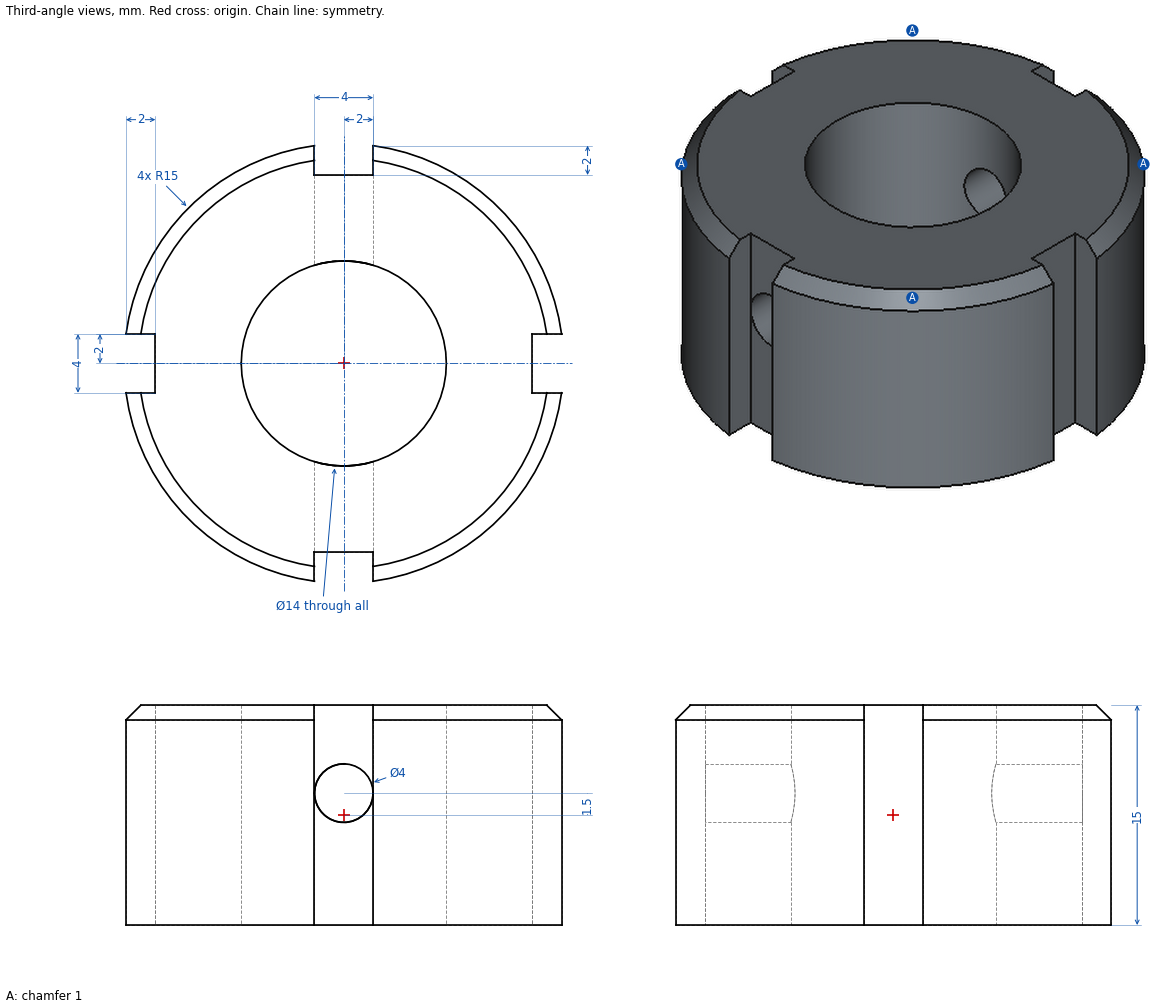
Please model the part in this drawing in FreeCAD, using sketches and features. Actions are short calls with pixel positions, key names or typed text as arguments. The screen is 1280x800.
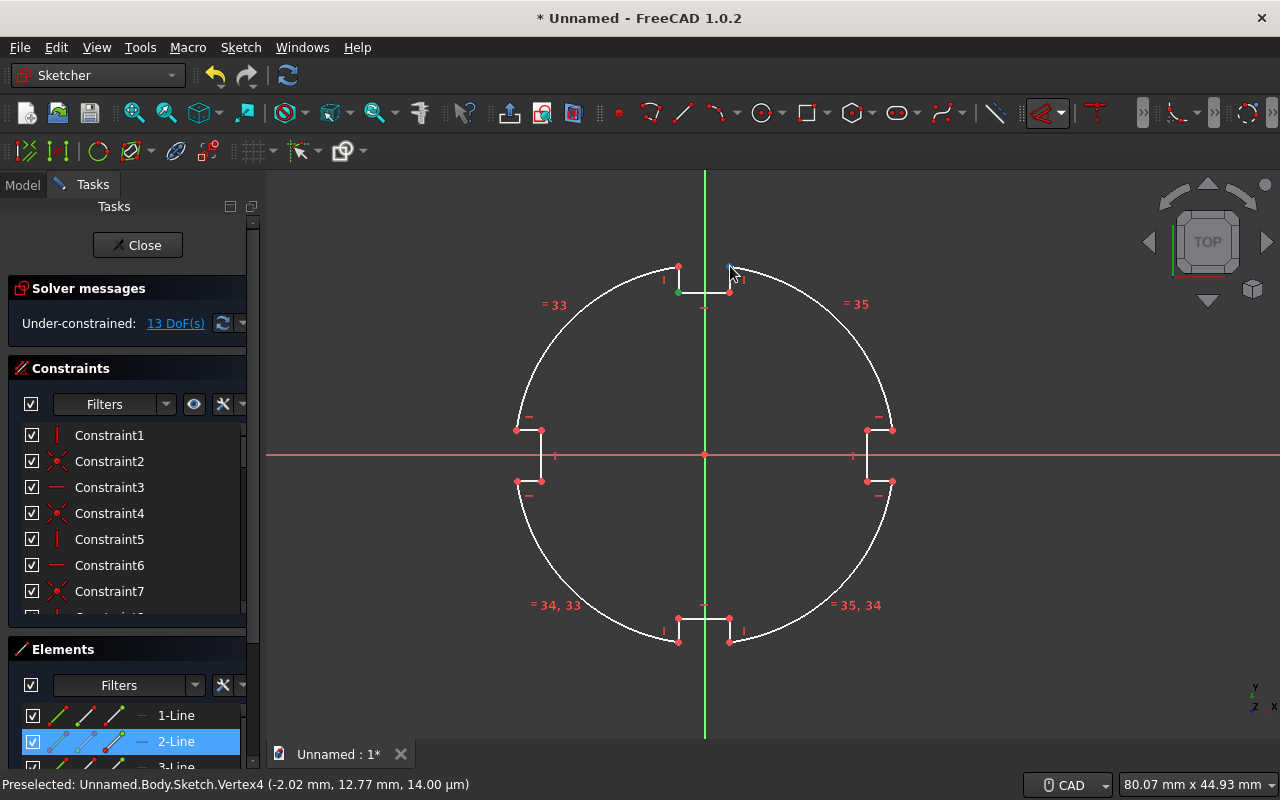
click(679, 619)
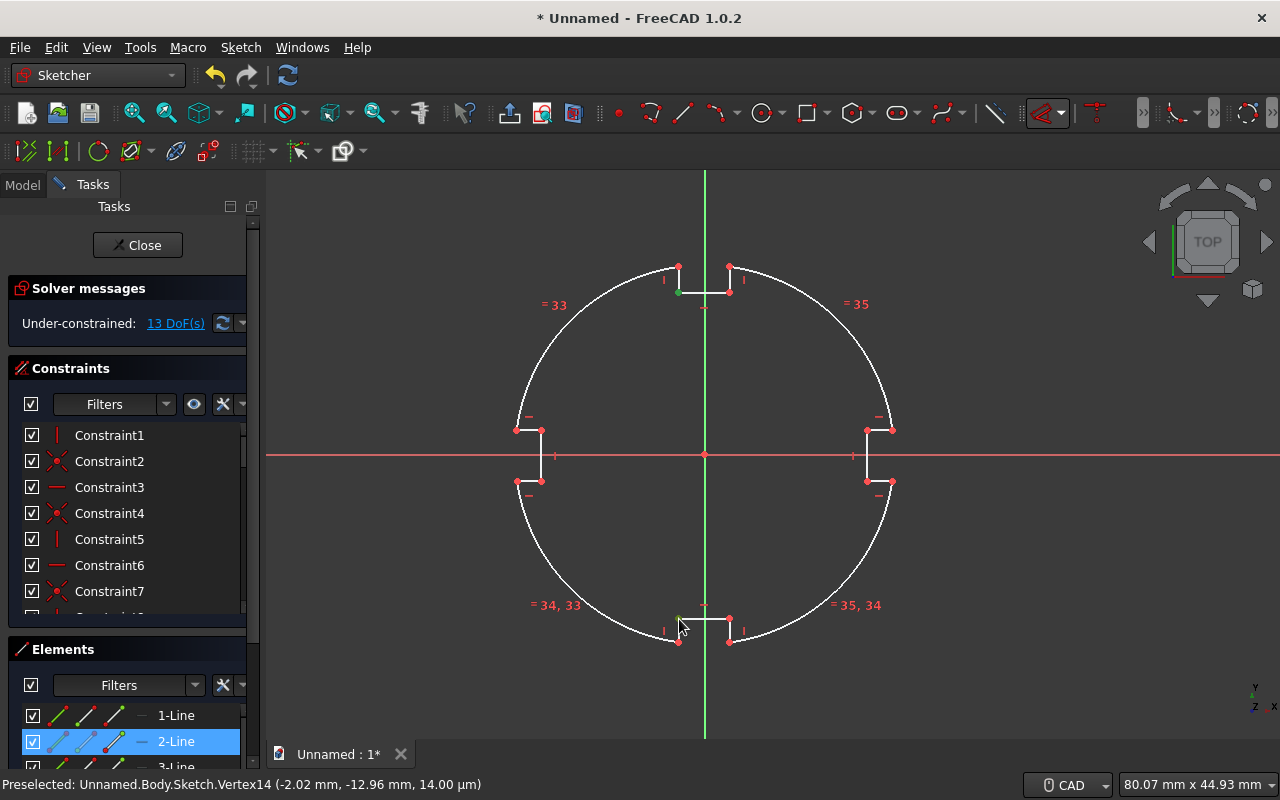
click(353, 455)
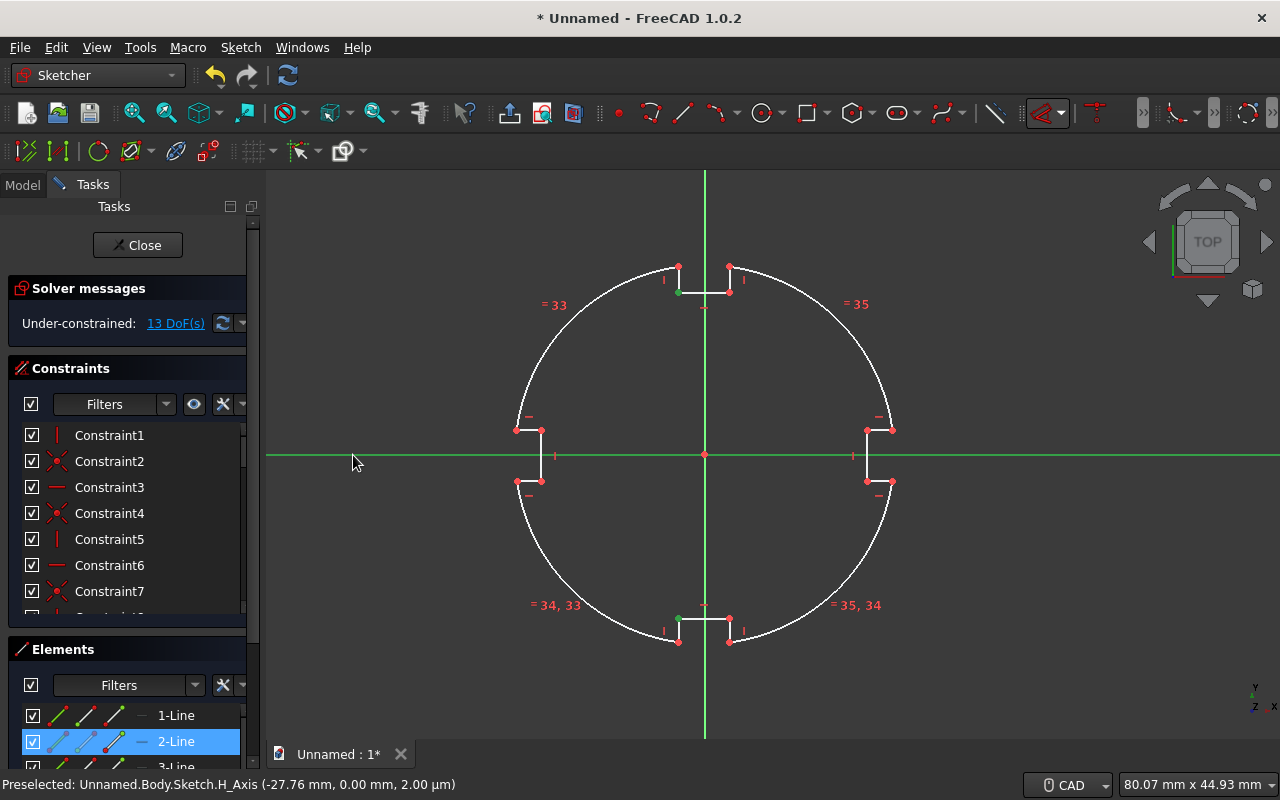
key(s)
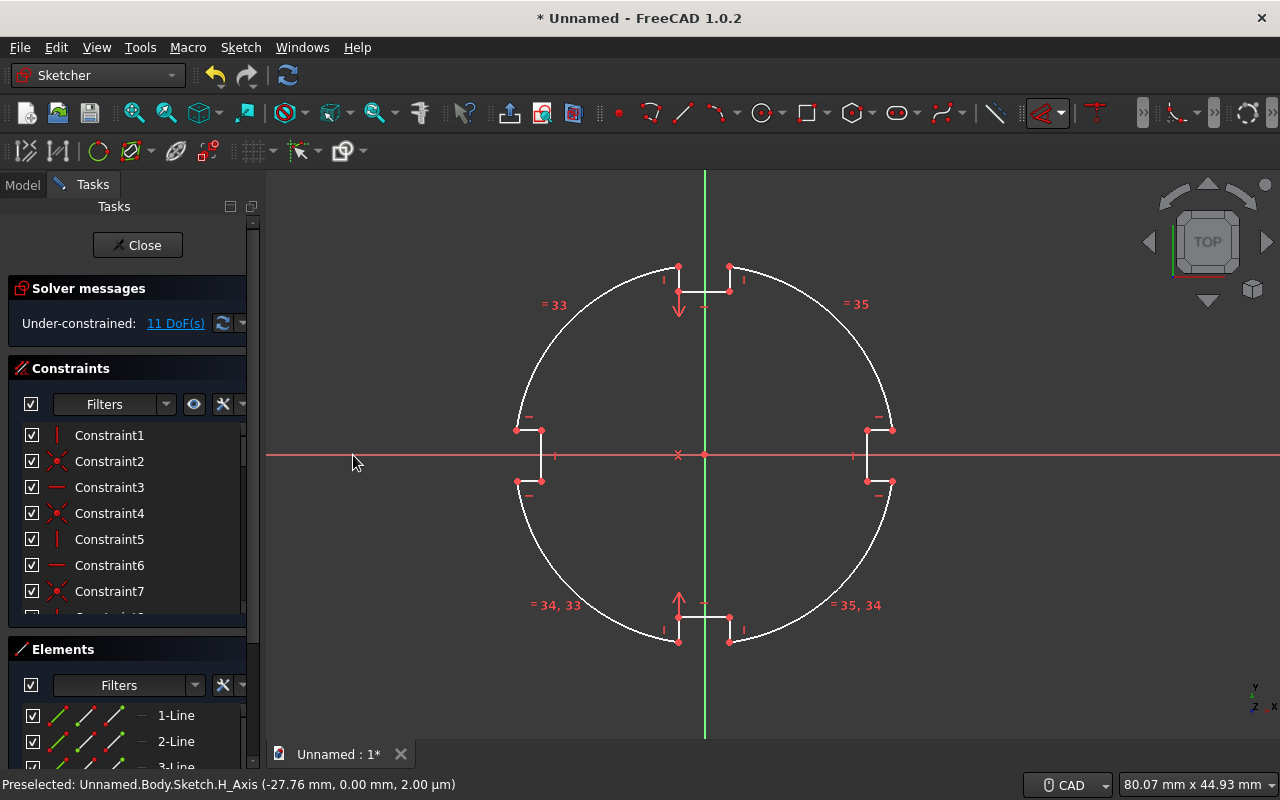
click(541, 481)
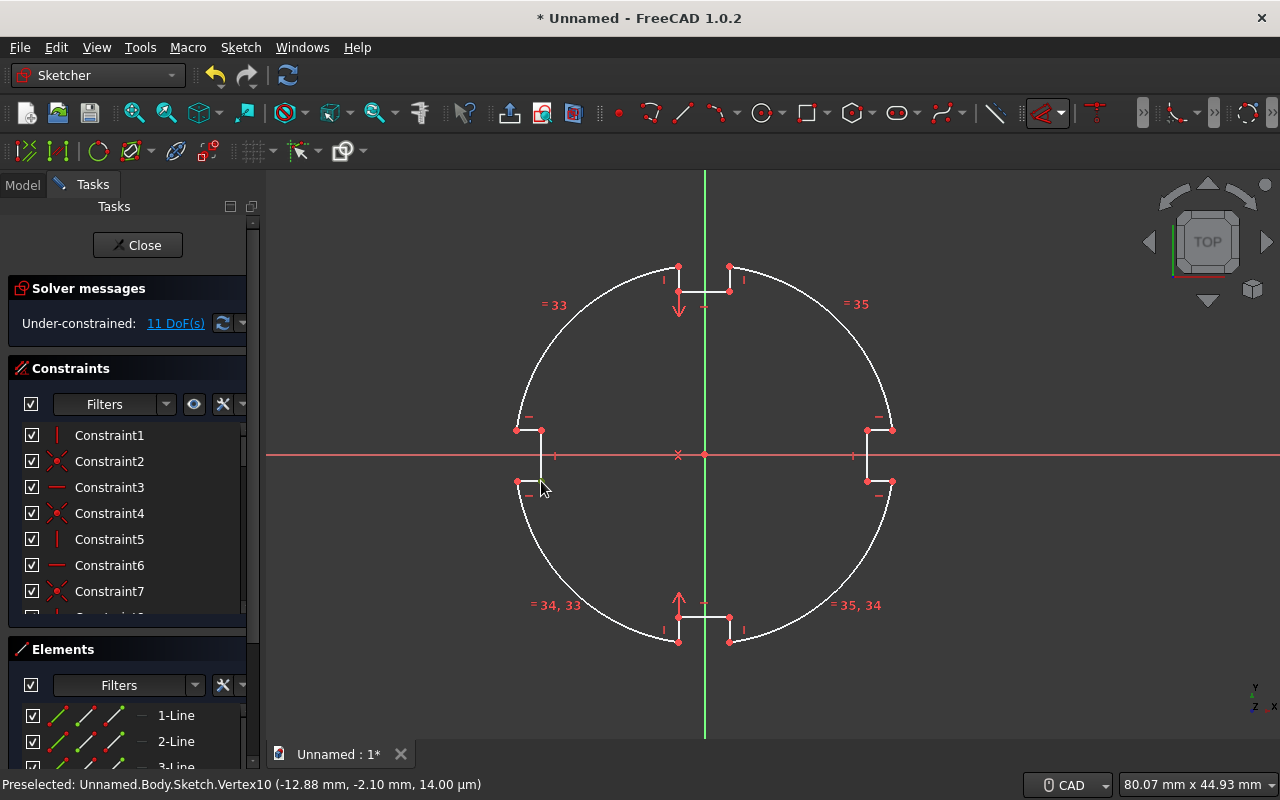
click(867, 481)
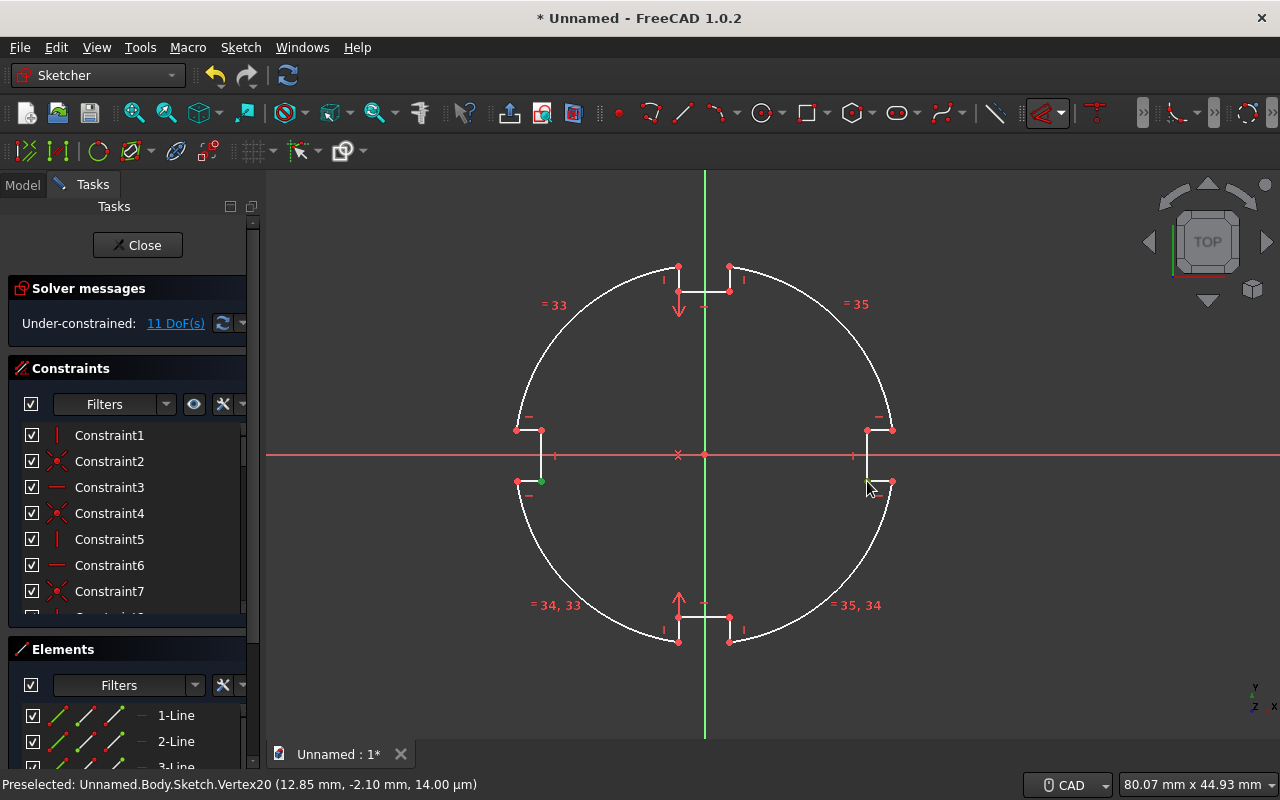
click(705, 674)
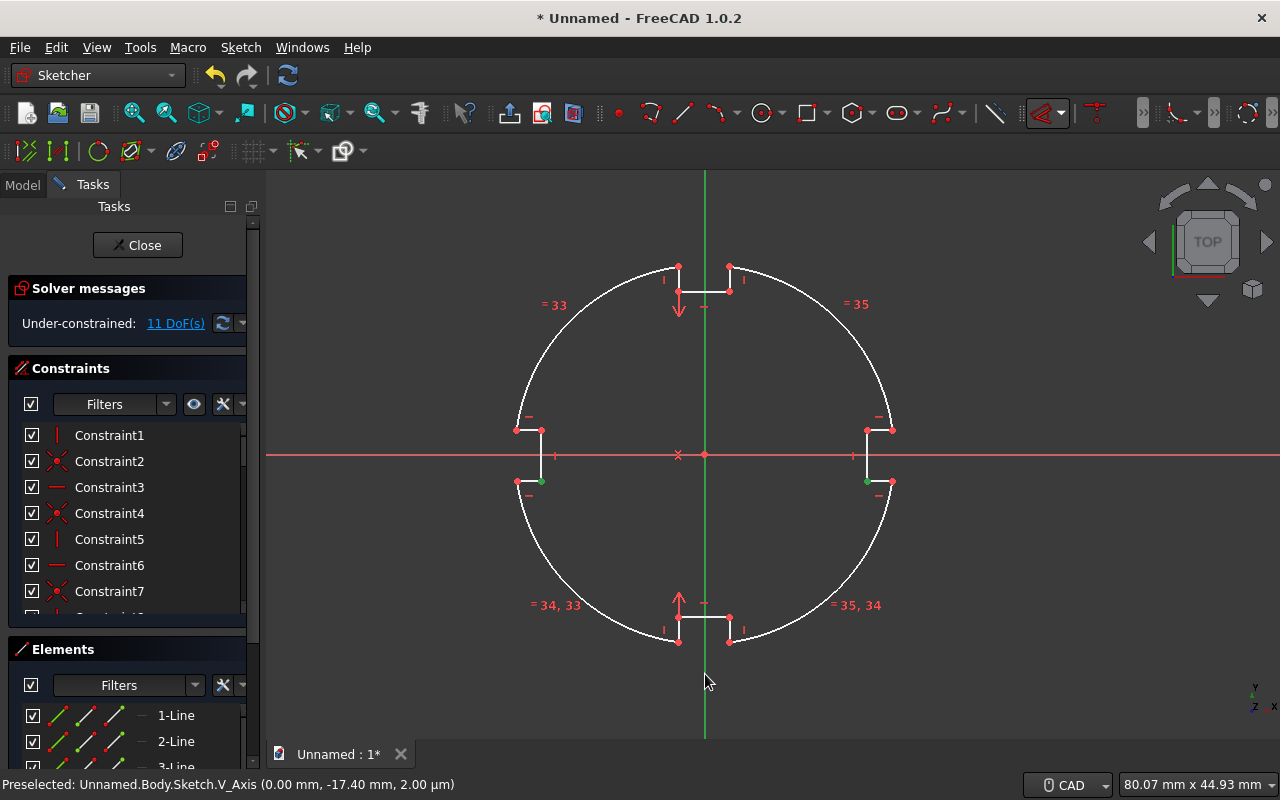
key(s)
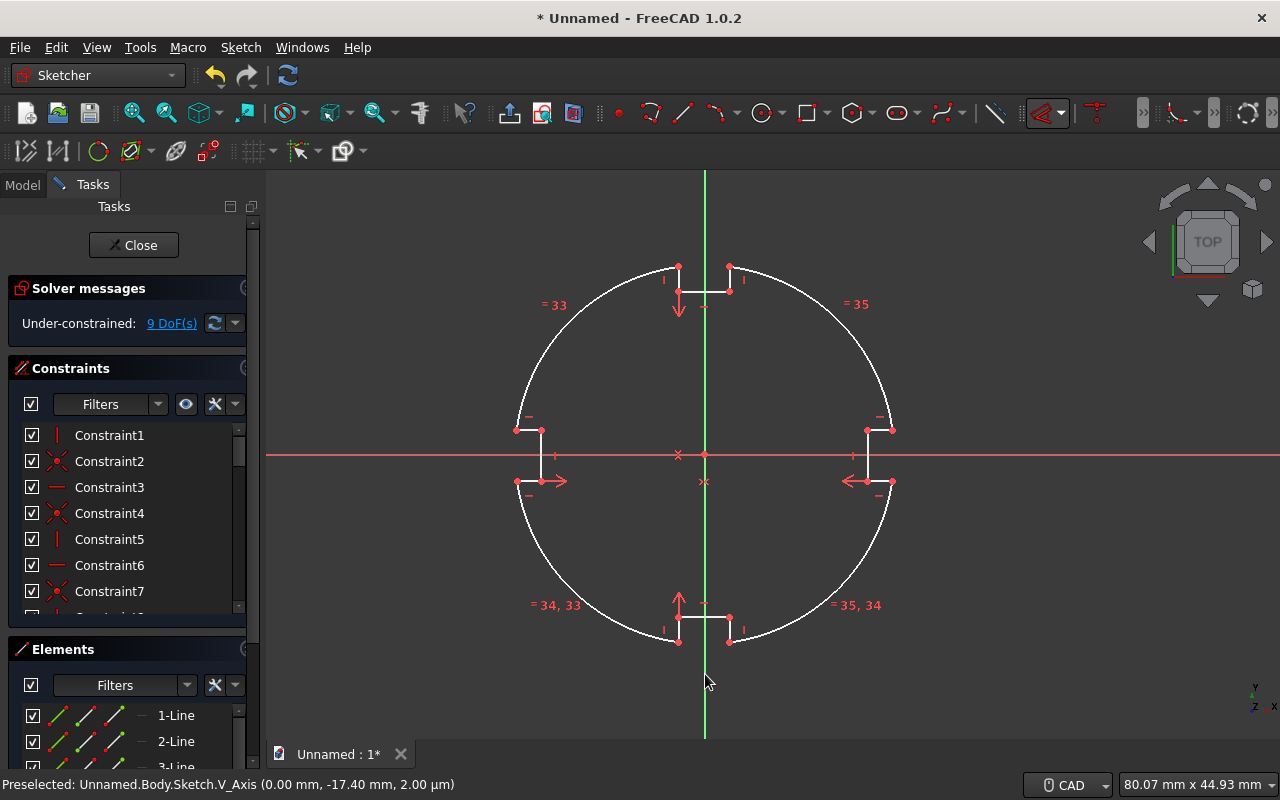
click(609, 291)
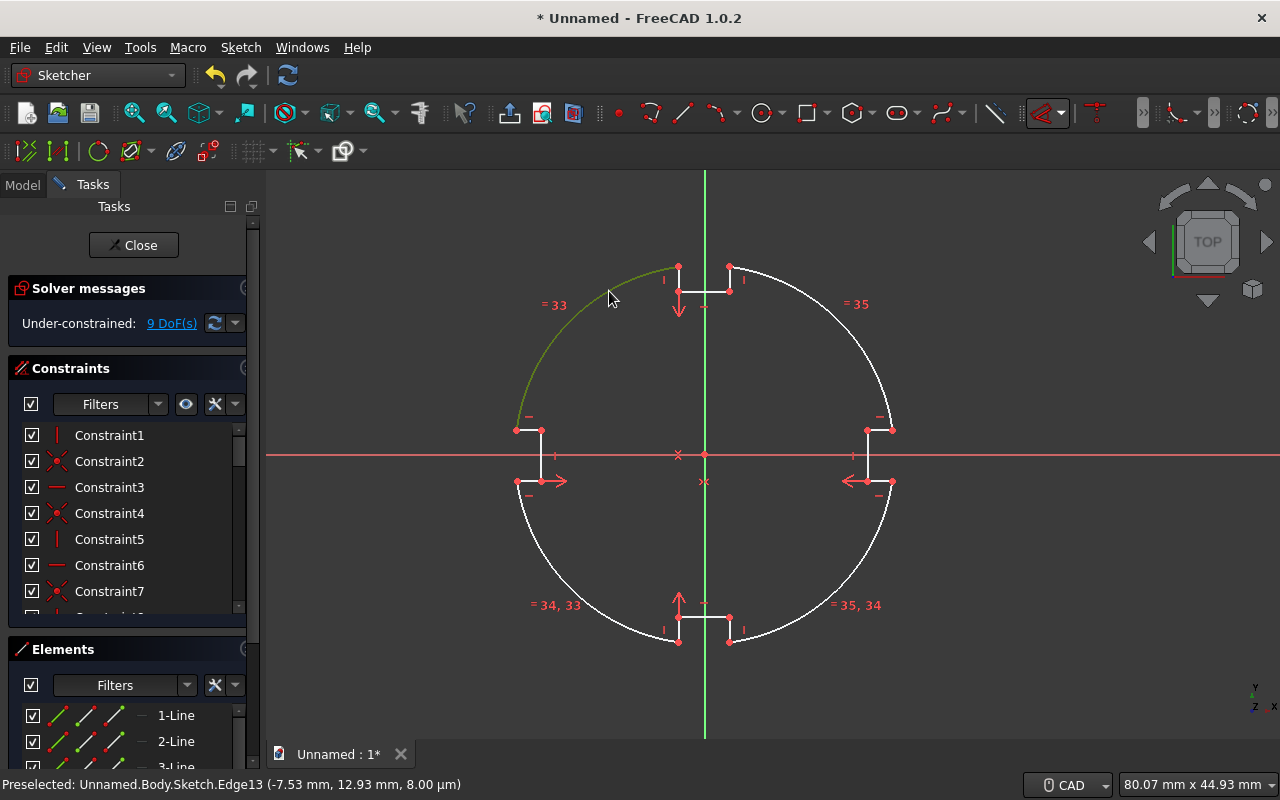
key(k)
key(r)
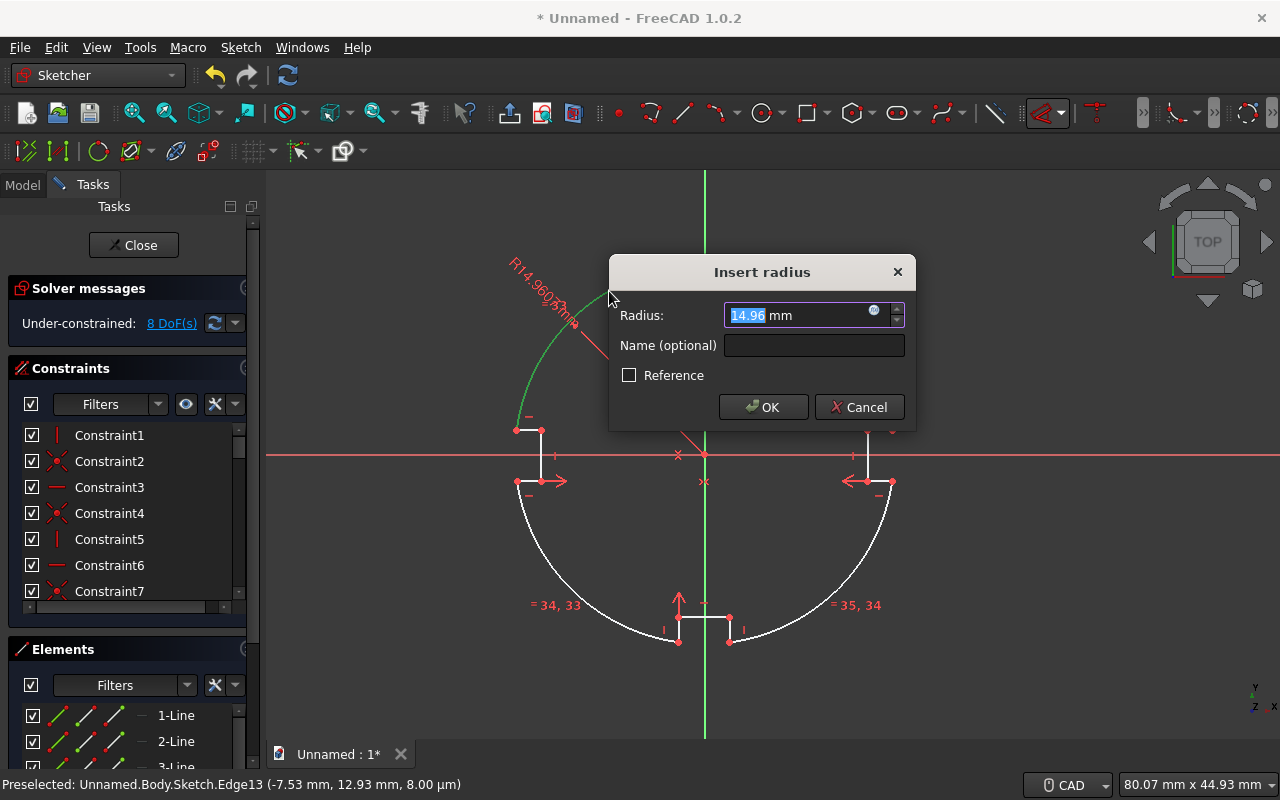
text(15)
key(Return)